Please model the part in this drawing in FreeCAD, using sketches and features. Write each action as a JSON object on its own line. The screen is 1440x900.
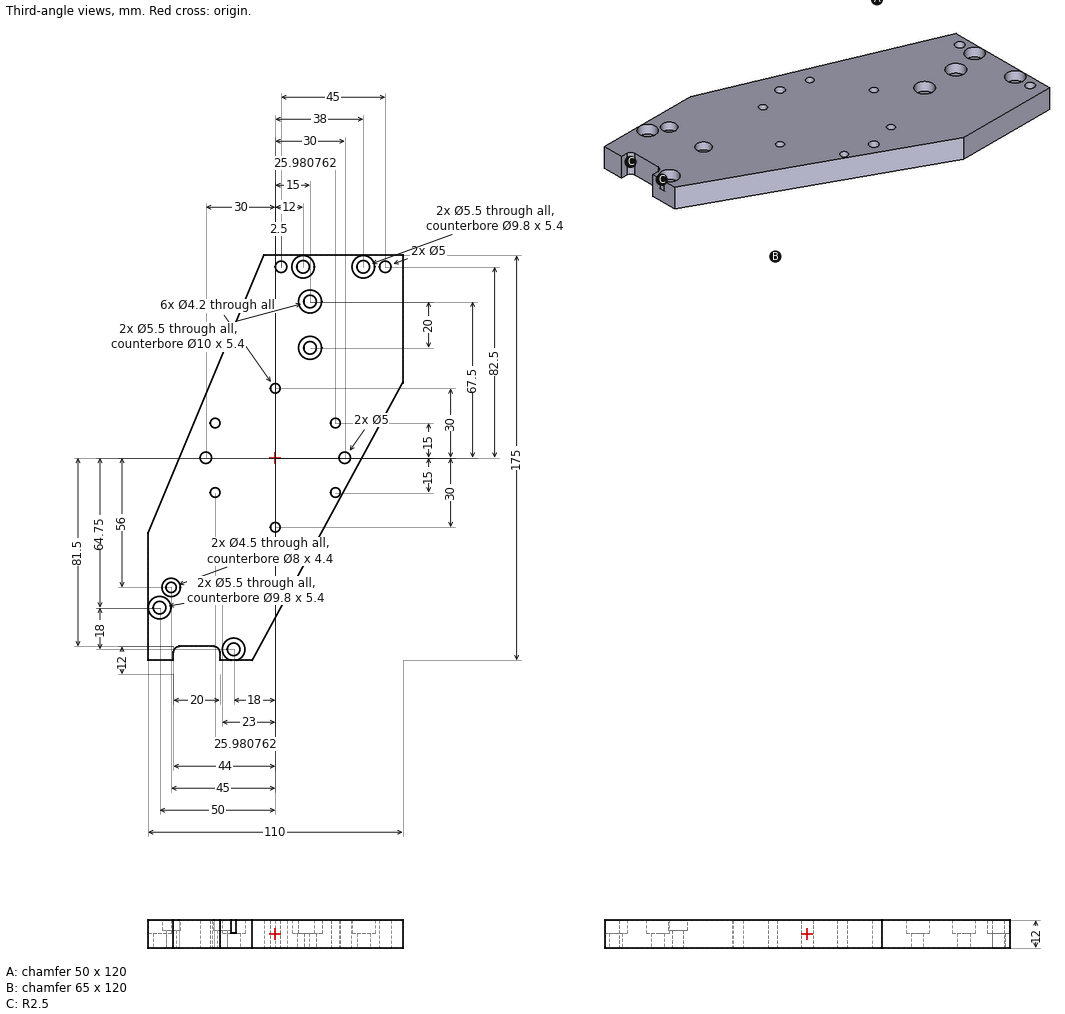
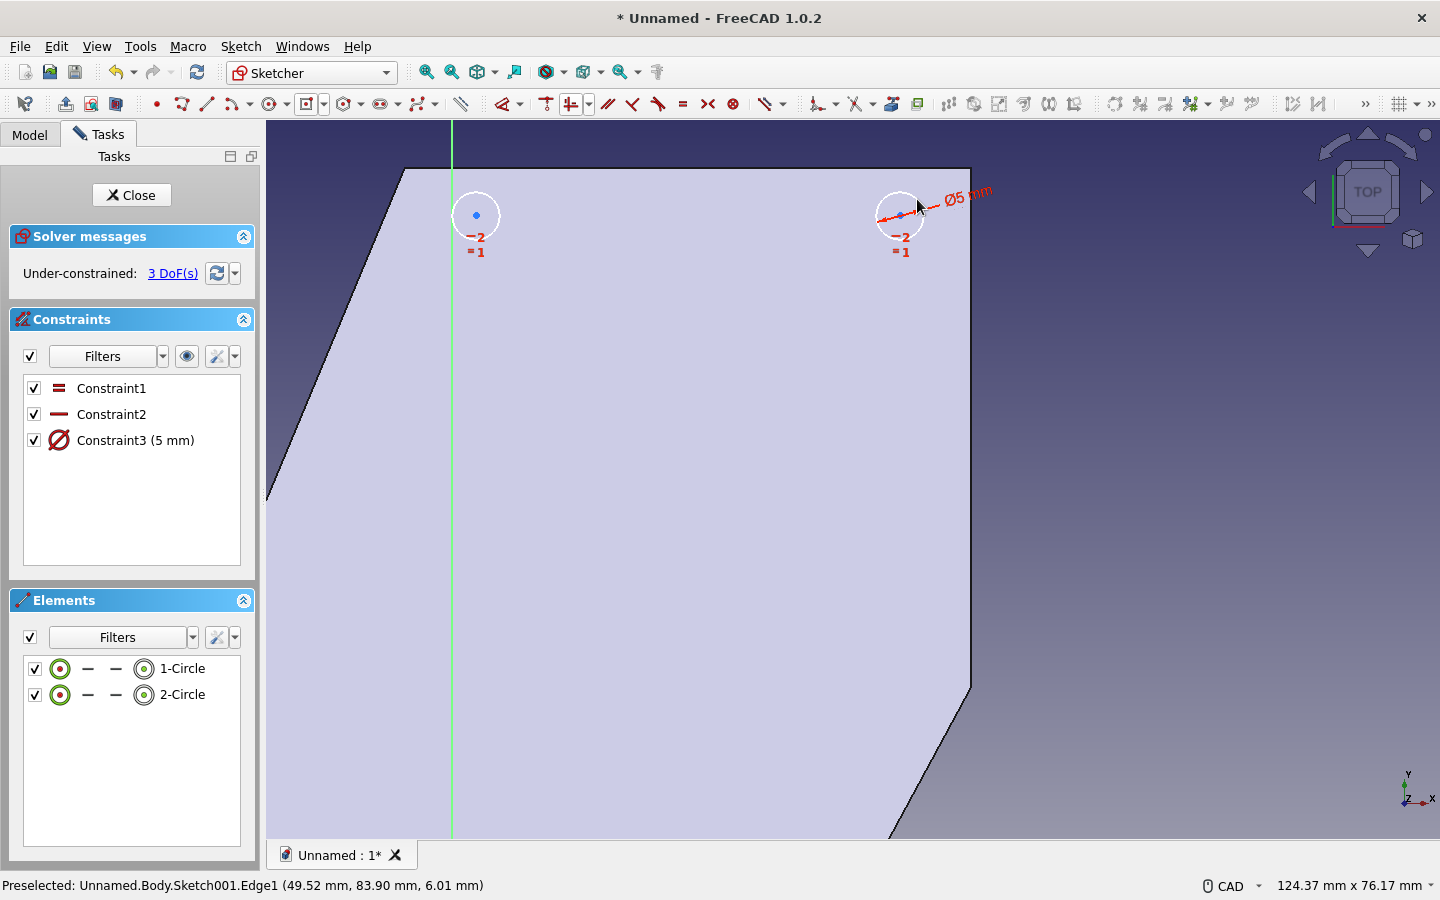
{"action": "scroll", "coordinate": [476, 216], "scroll_direction": "up", "scroll_amount": 3}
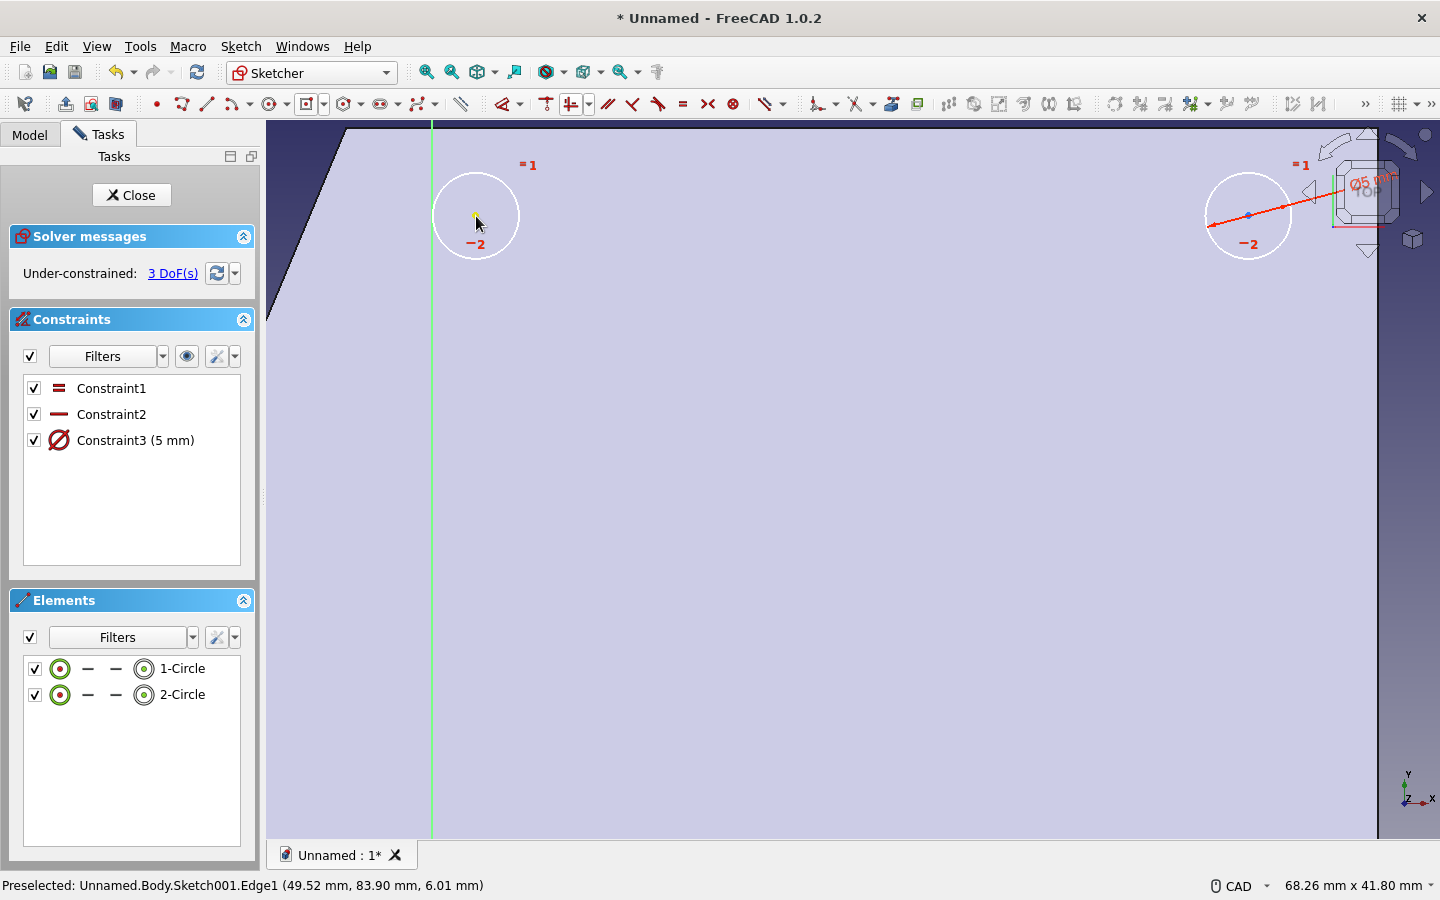
{"action": "left_click", "coordinate": [476, 216]}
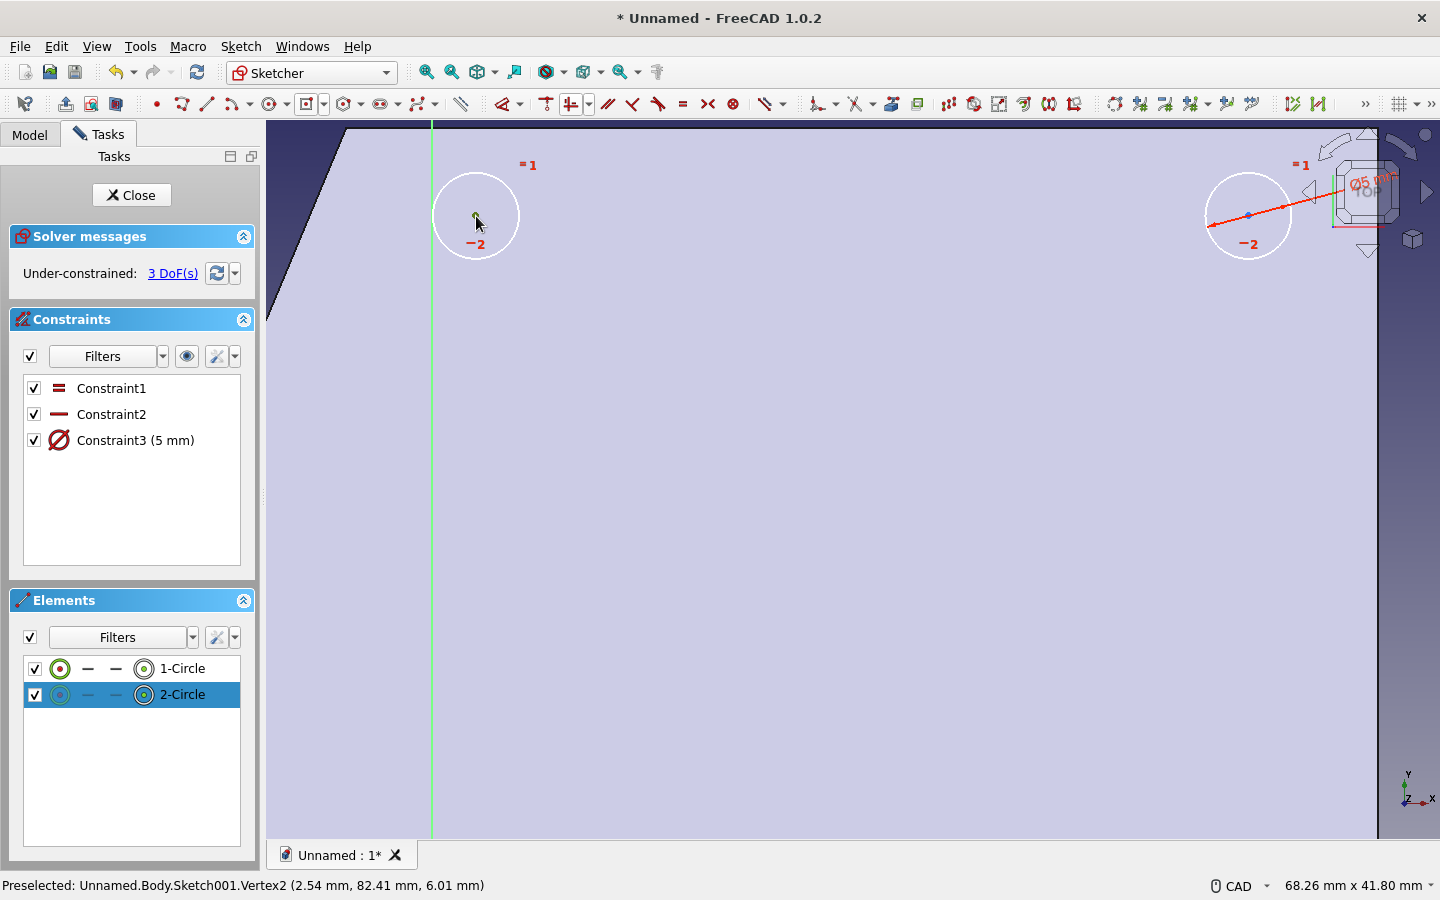
{"action": "key", "text": "l"}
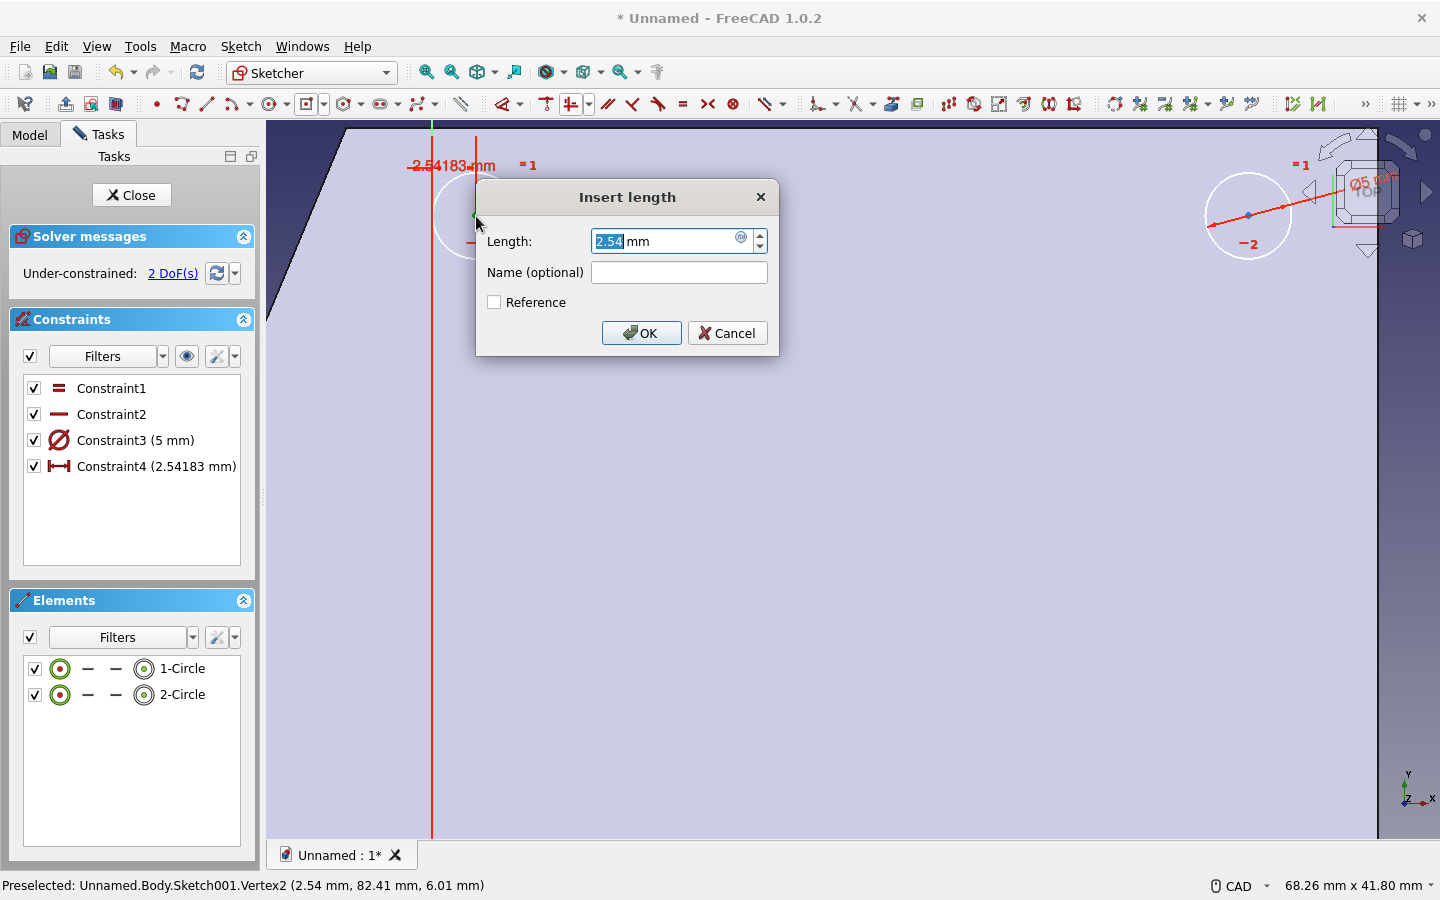
{"action": "type", "text": "2.5"}
{"action": "key", "text": "Return"}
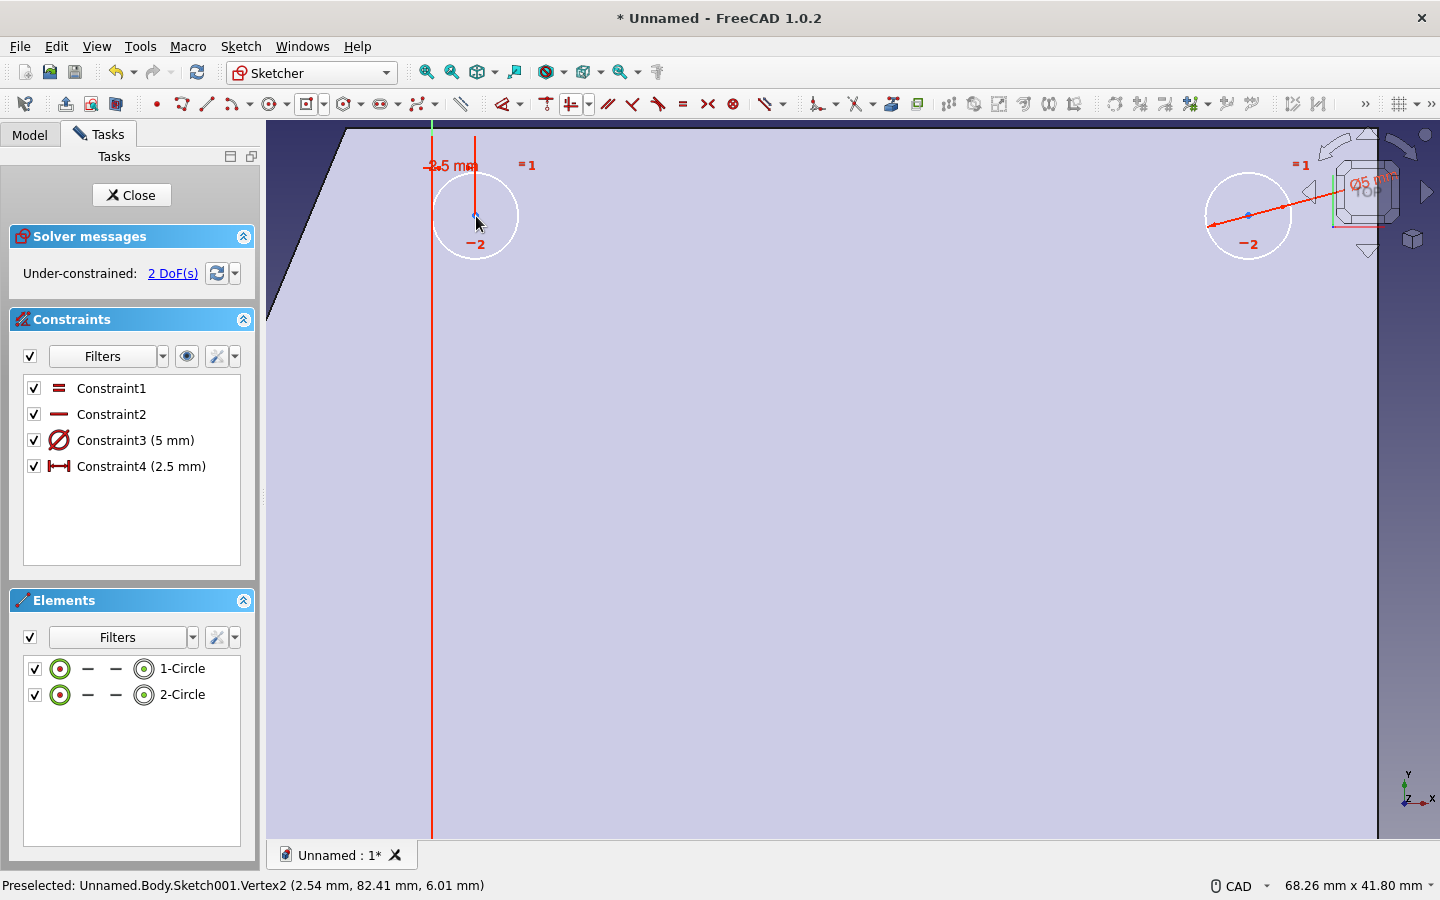
{"action": "left_click", "coordinate": [1248, 216]}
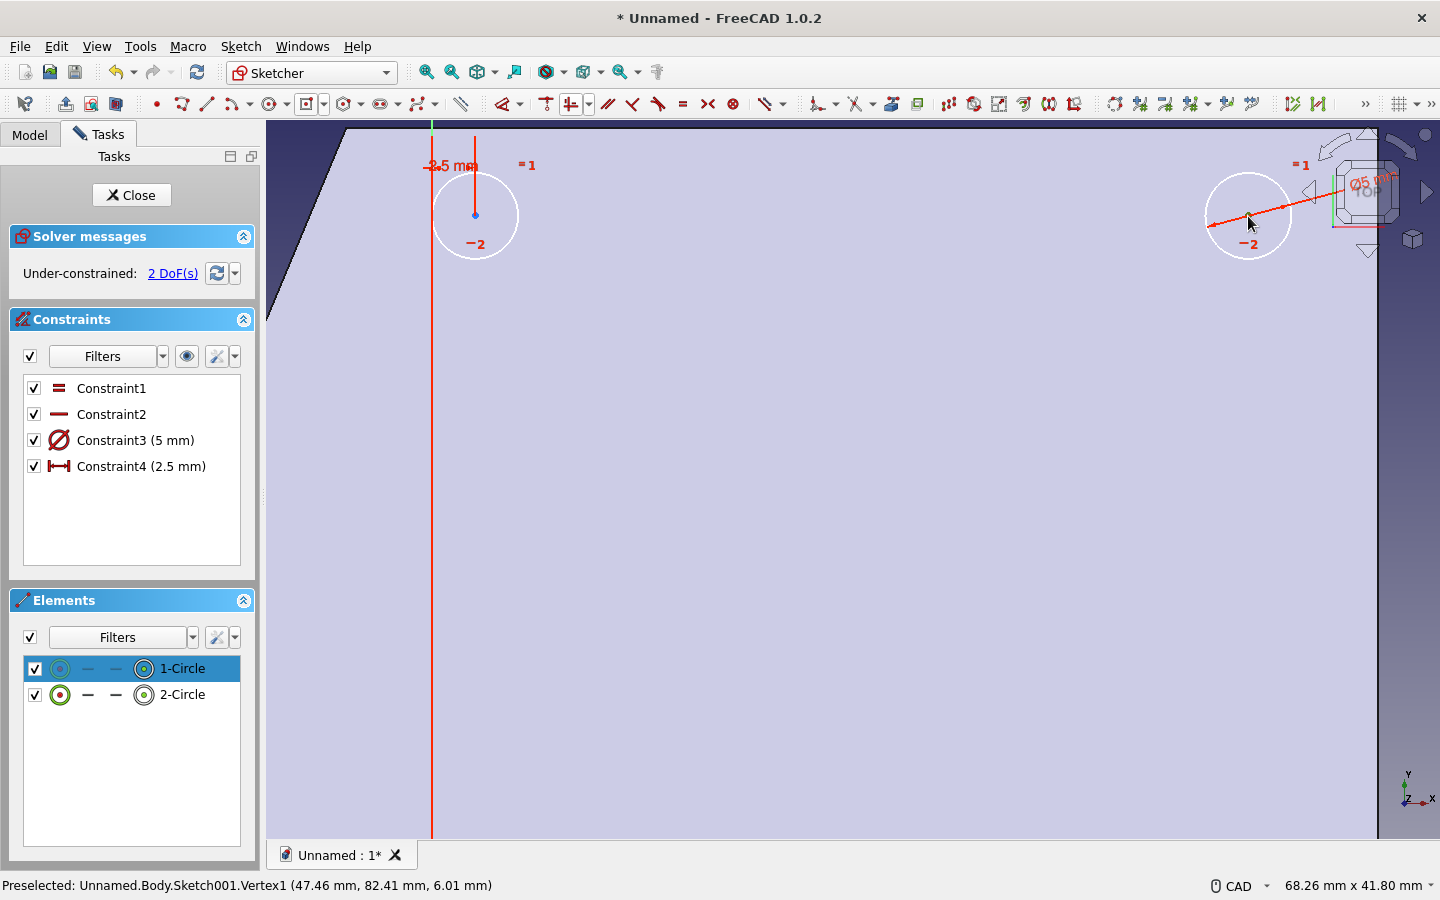
{"action": "left_click", "coordinate": [475, 216]}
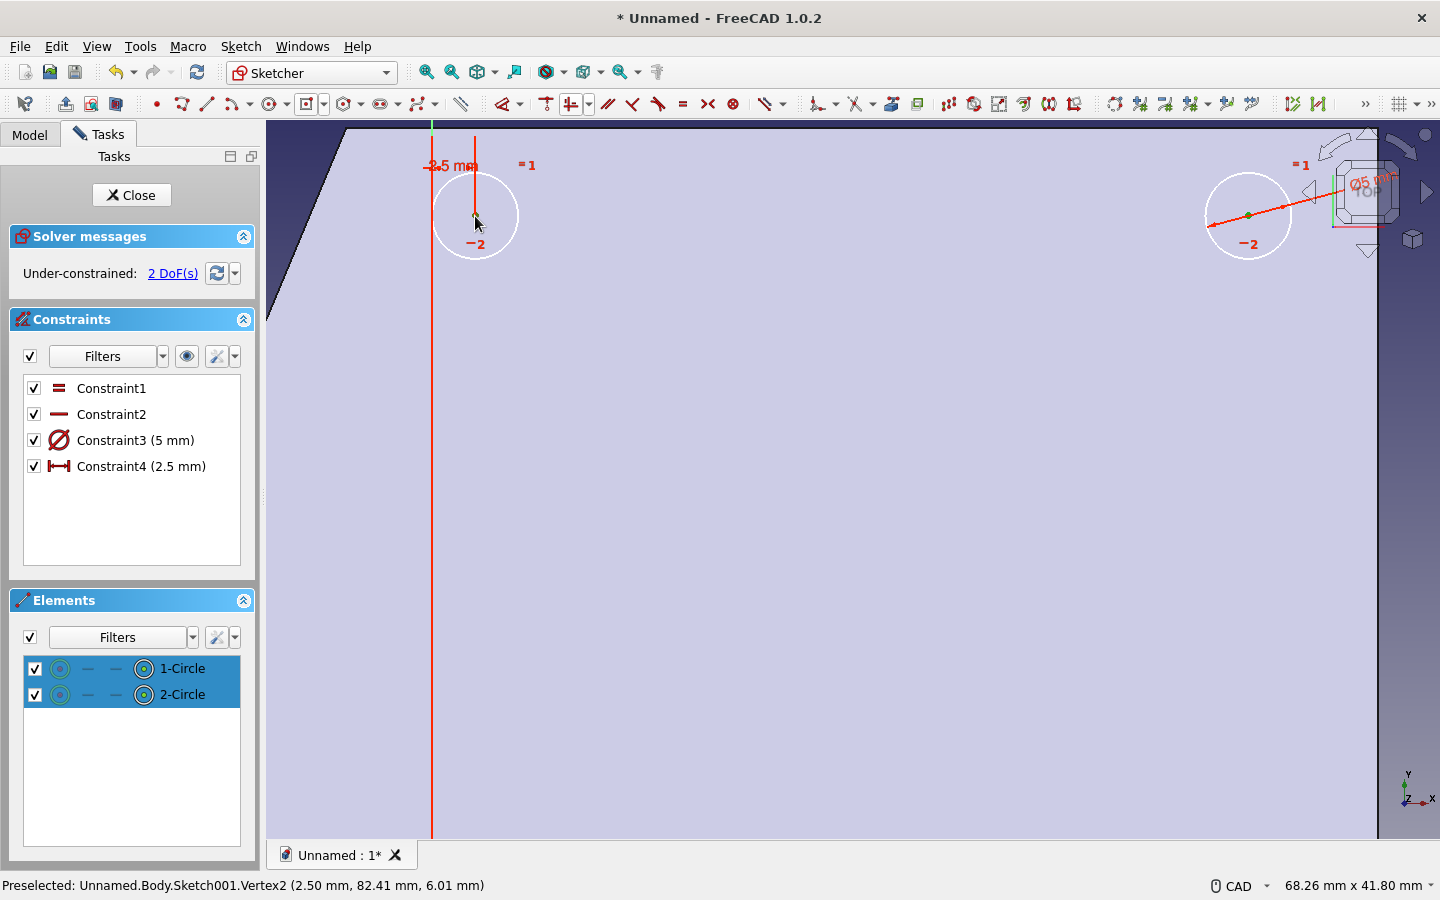
{"action": "key", "text": "l"}